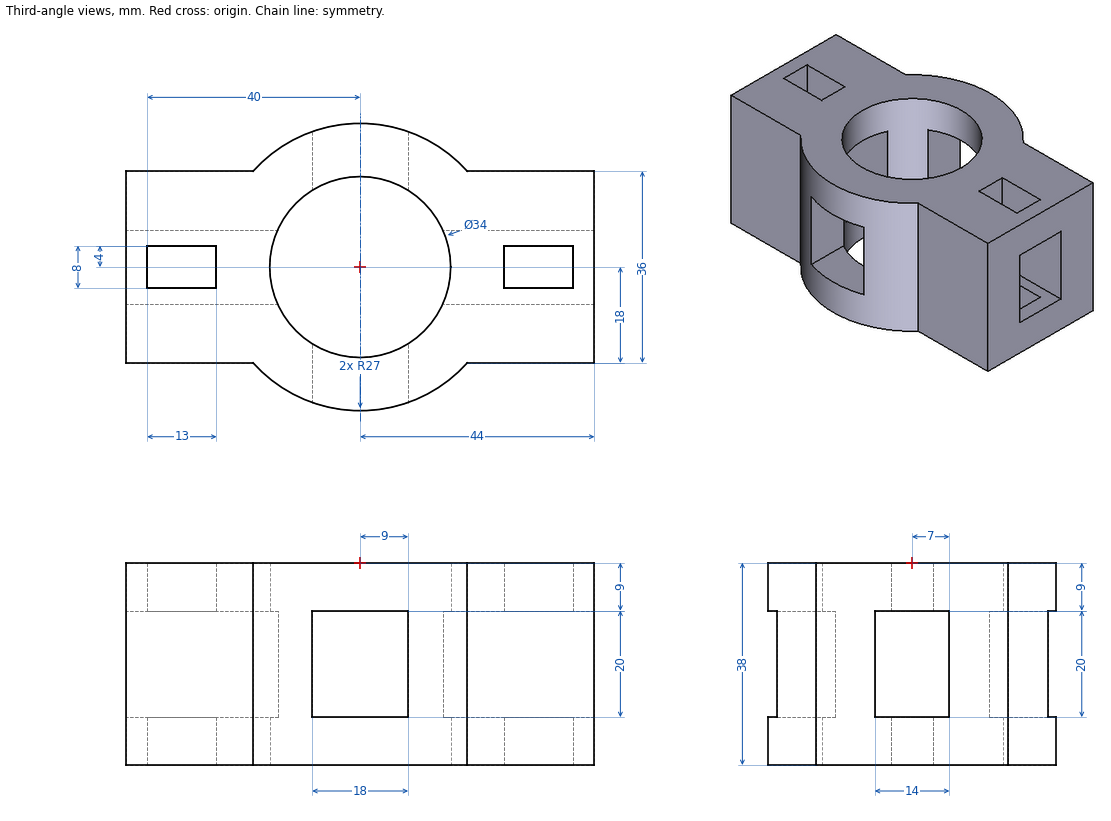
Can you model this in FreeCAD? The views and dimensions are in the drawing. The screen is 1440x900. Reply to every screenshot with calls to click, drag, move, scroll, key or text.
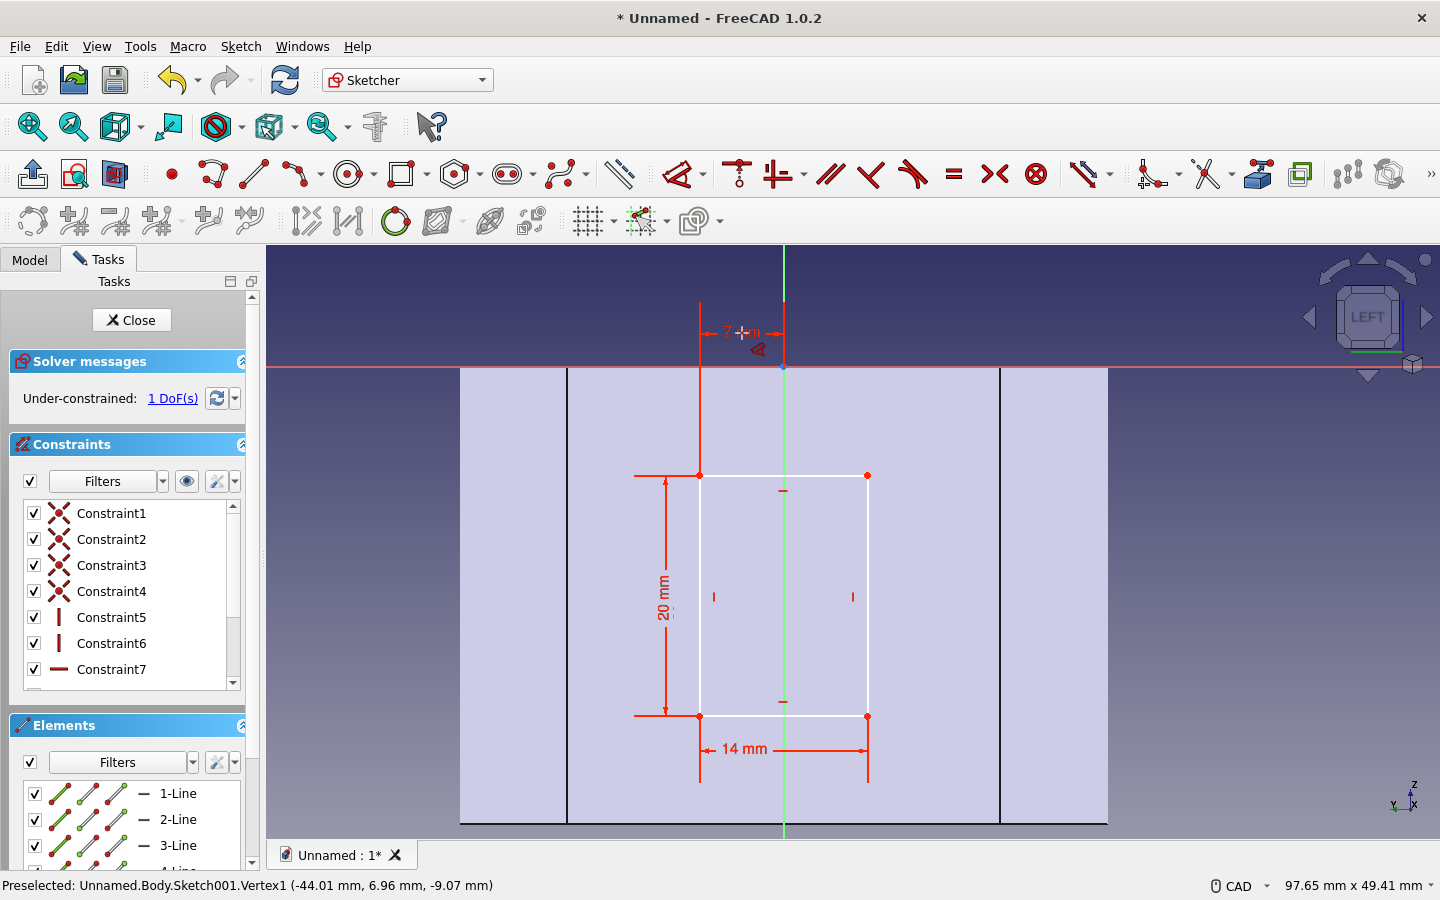
click(700, 476)
click(666, 421)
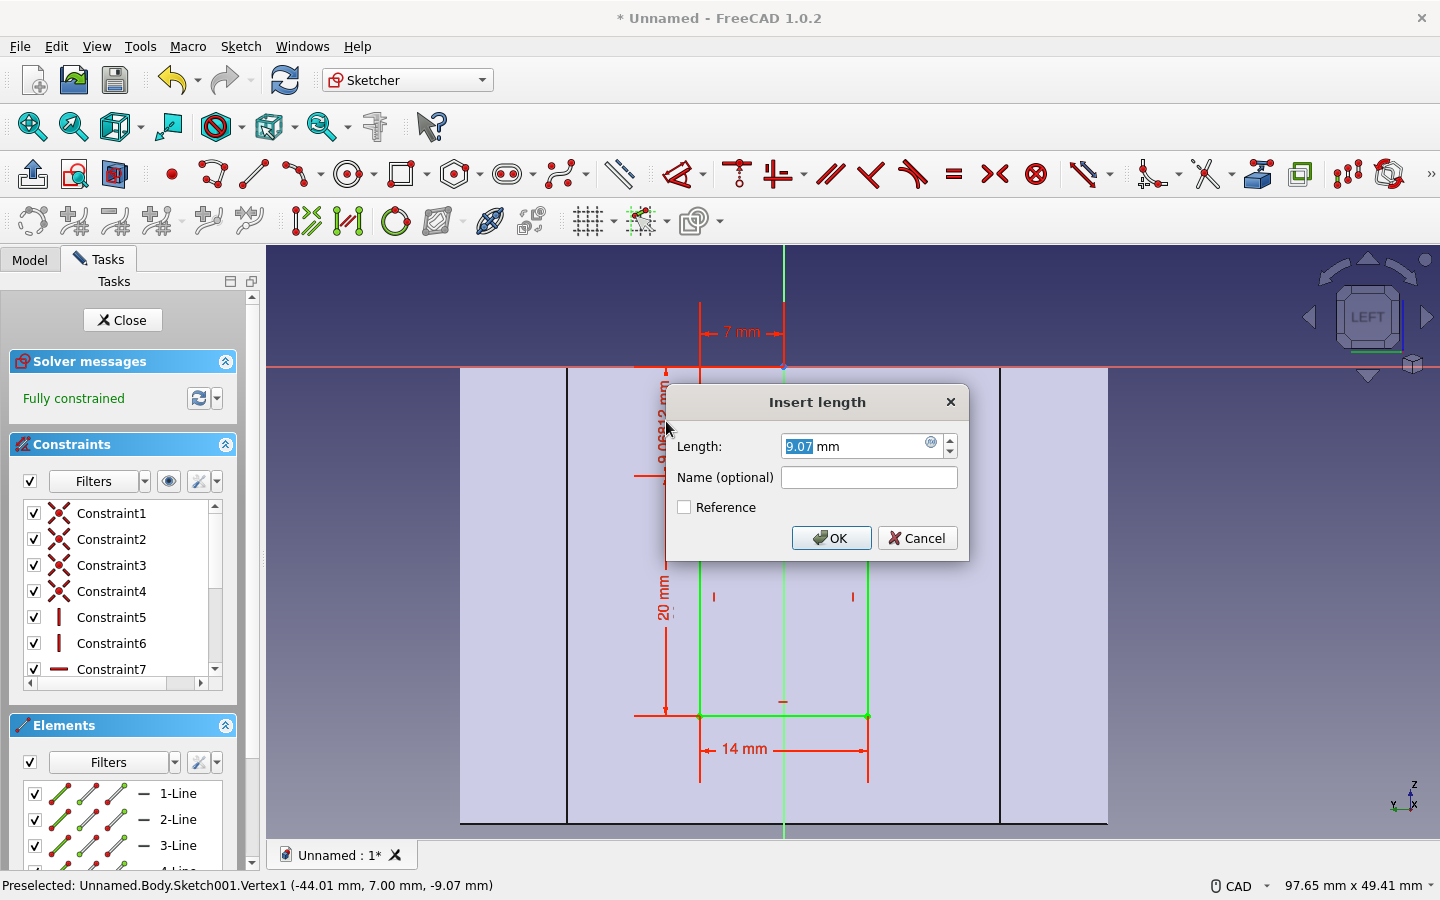
text(9)
key(Return)
key(Escape)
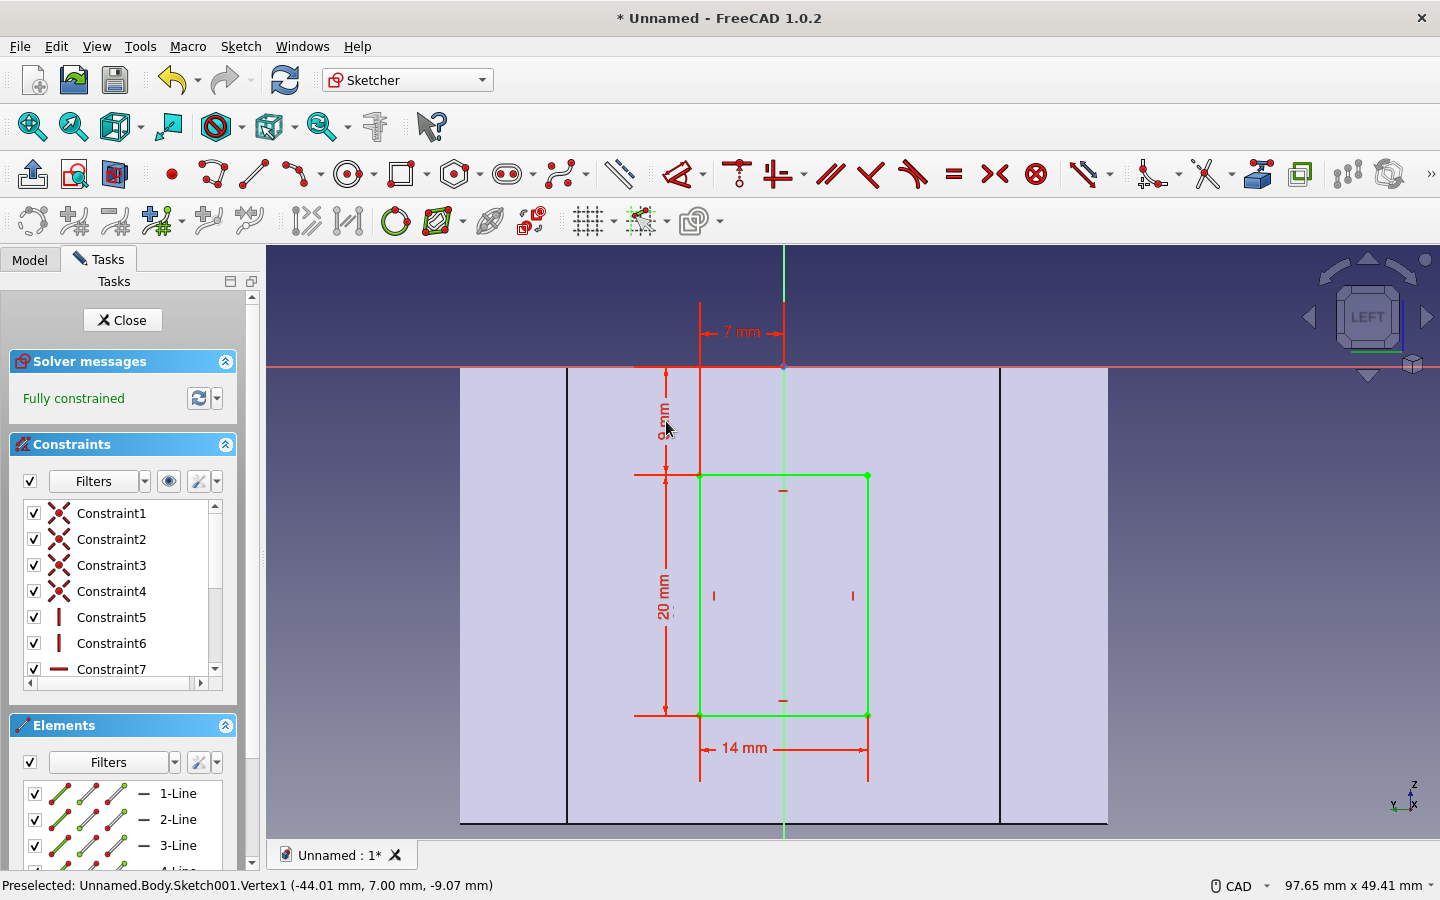
click(123, 320)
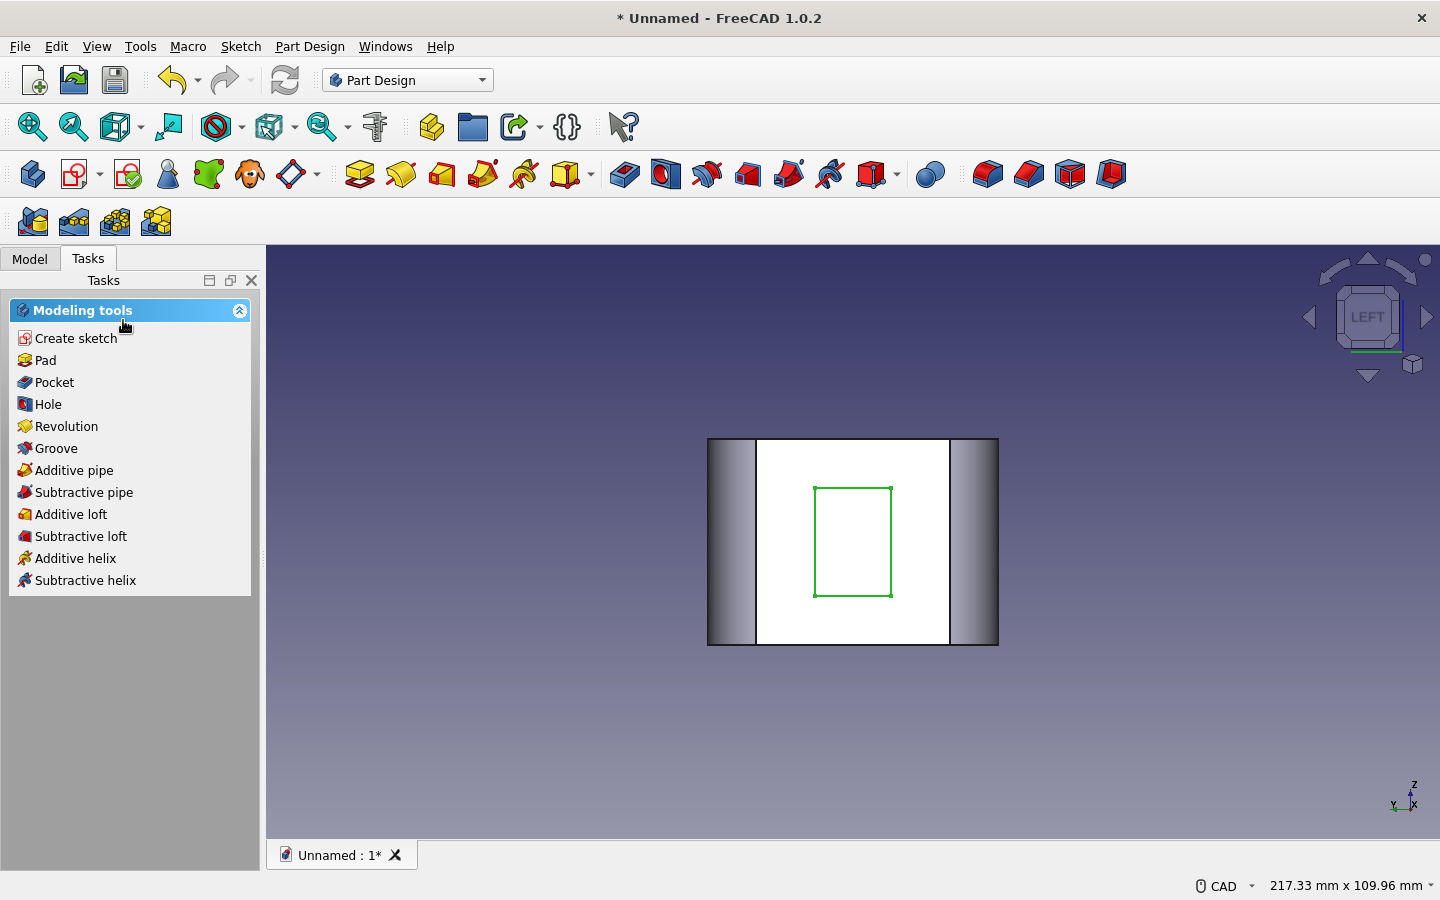
click(625, 174)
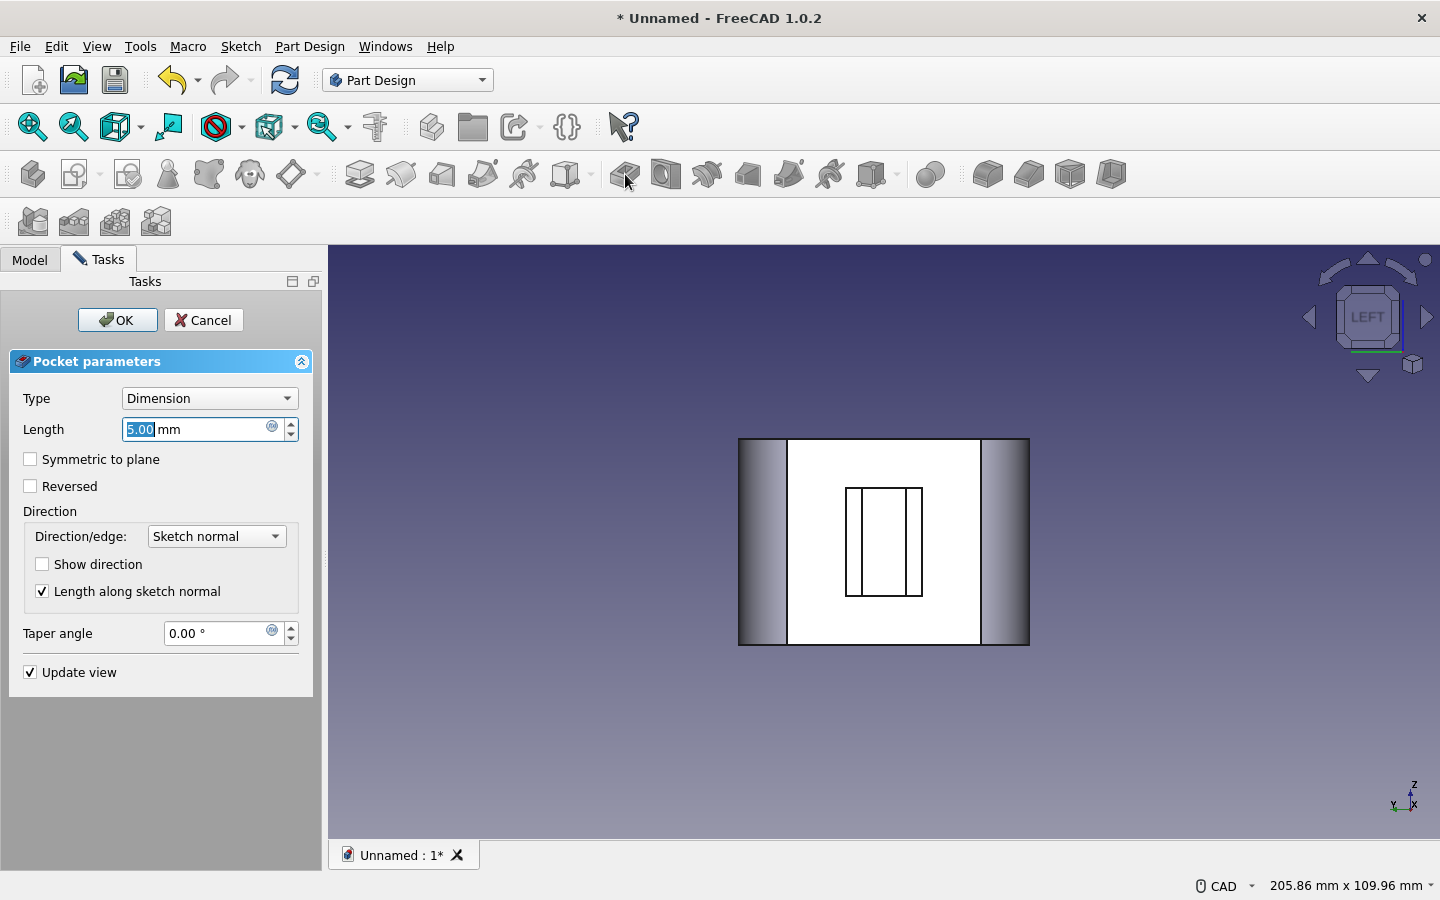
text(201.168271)
key(Tab)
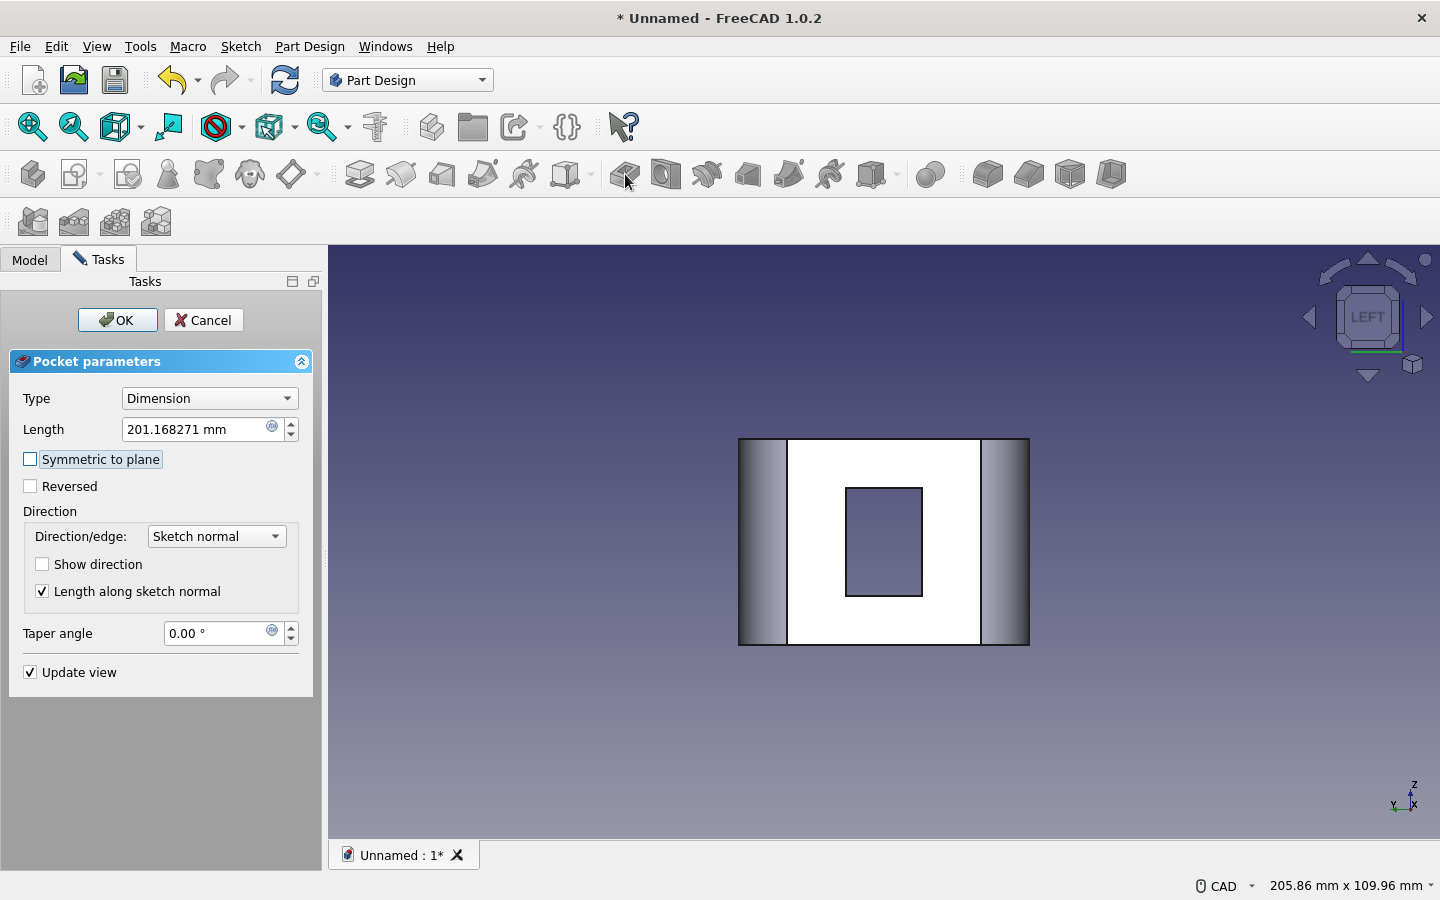
click(31, 459)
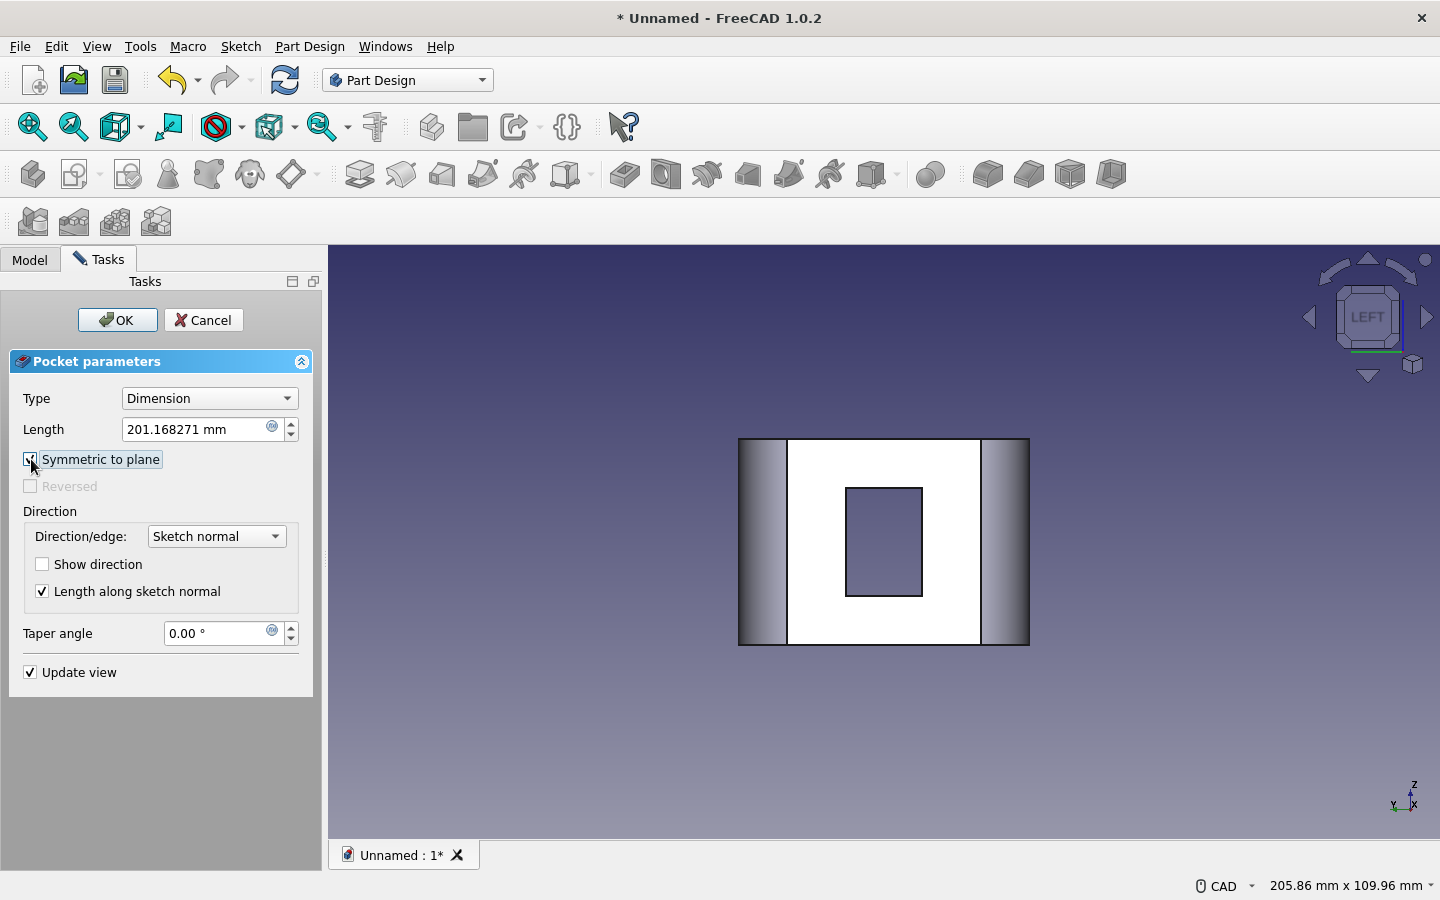
click(118, 320)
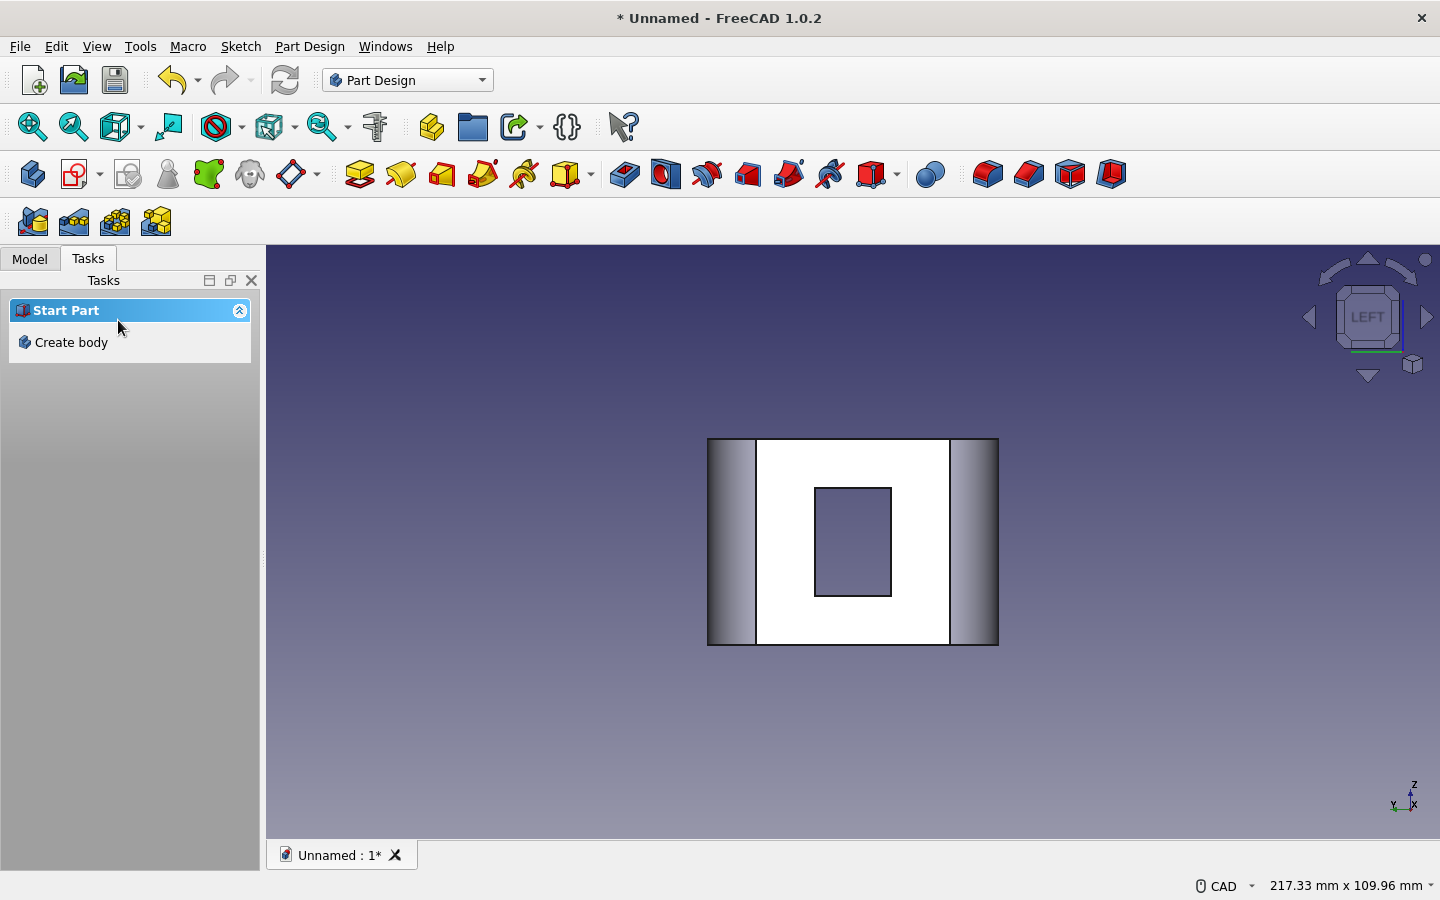
click(33, 128)